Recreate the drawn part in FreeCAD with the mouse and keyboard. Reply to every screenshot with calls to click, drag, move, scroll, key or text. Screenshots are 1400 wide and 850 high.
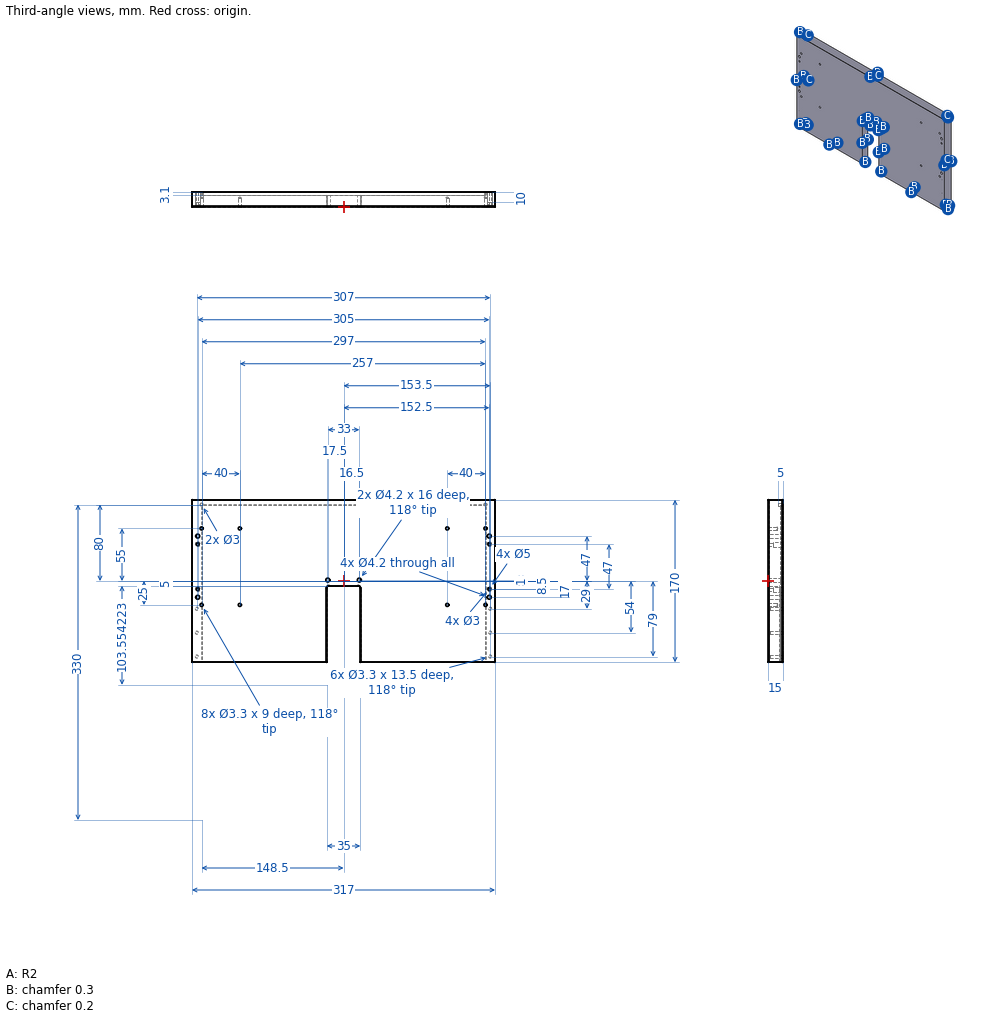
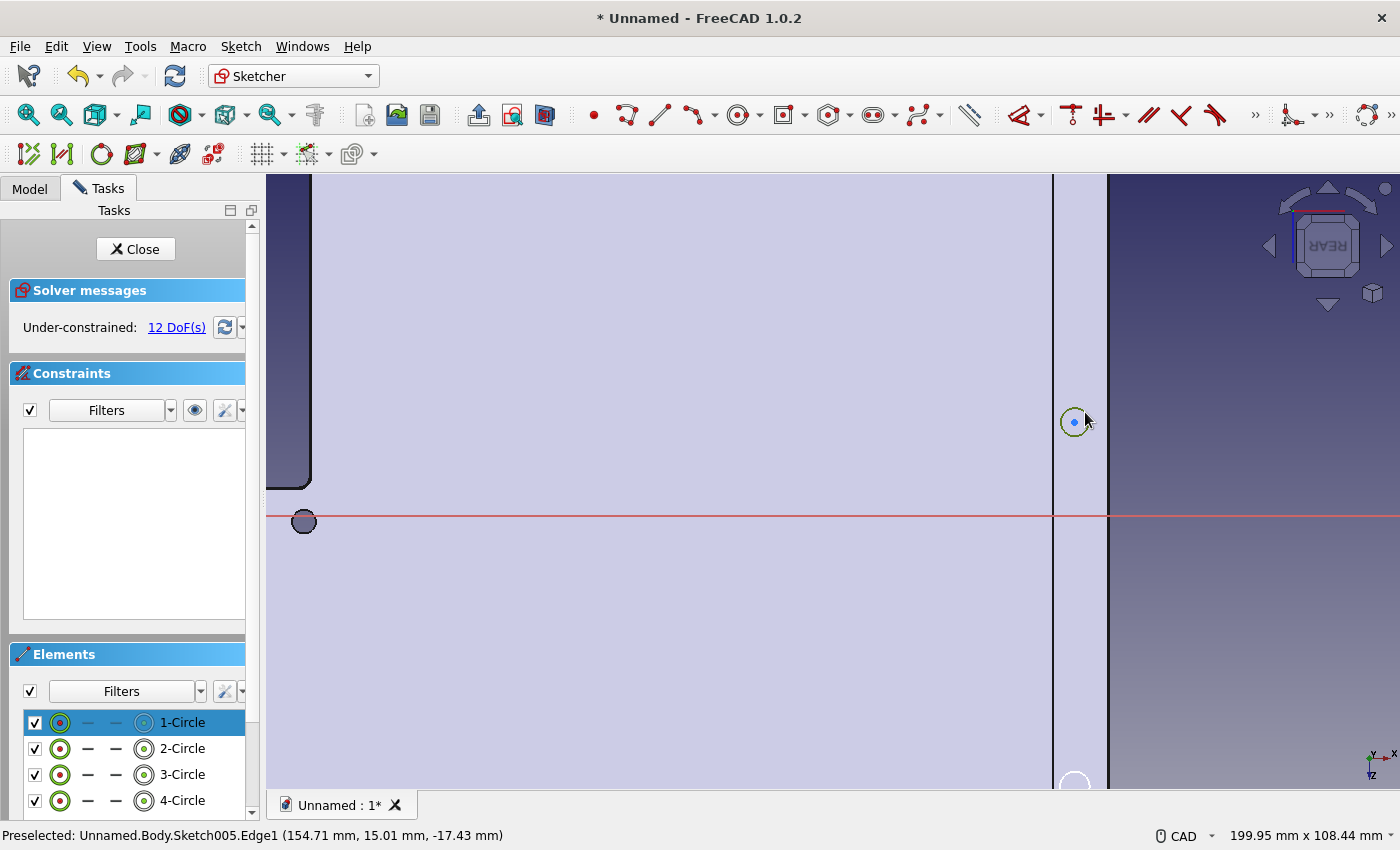
scroll(1087, 412, down, 5)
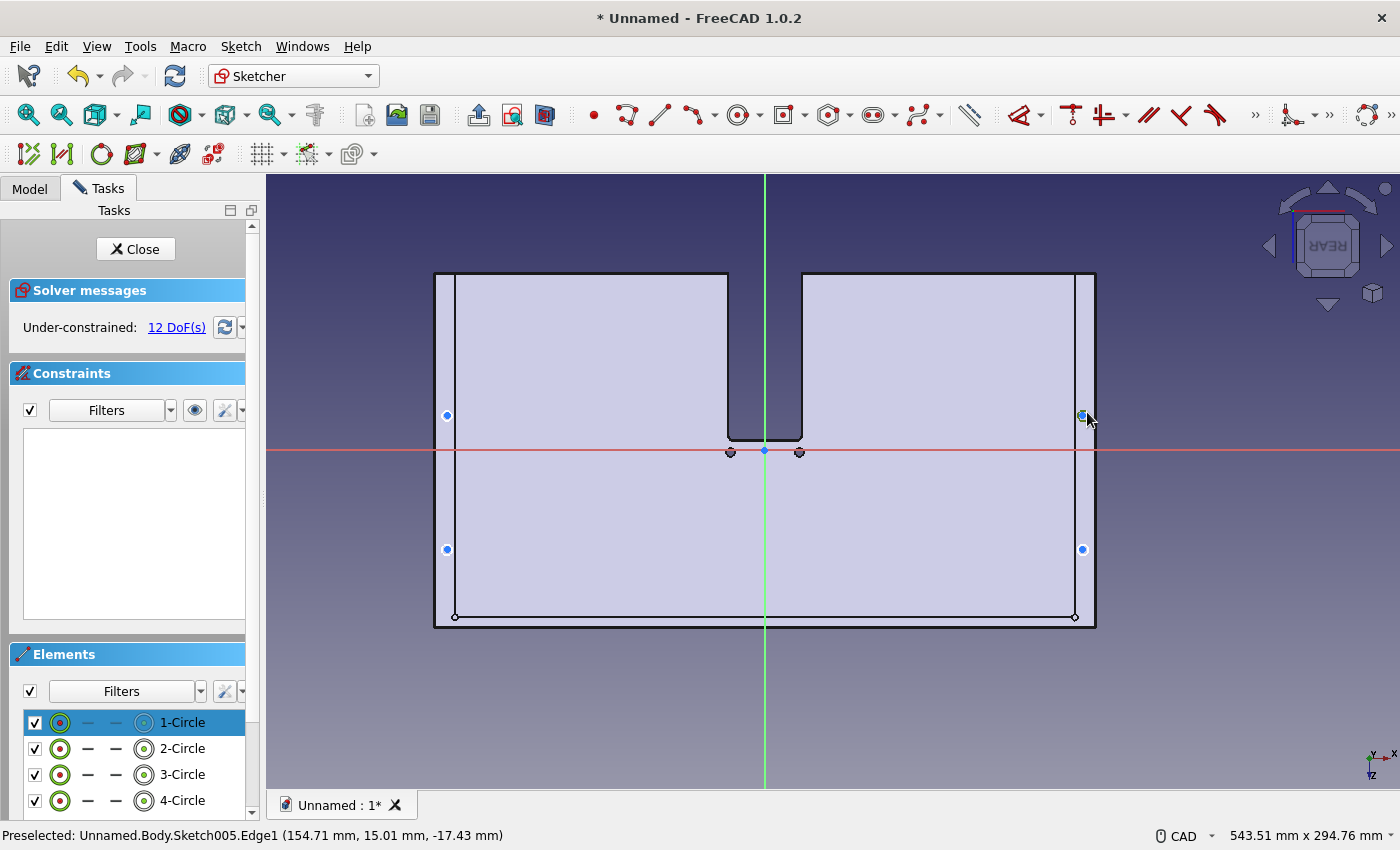
scroll(1087, 546, up, 5)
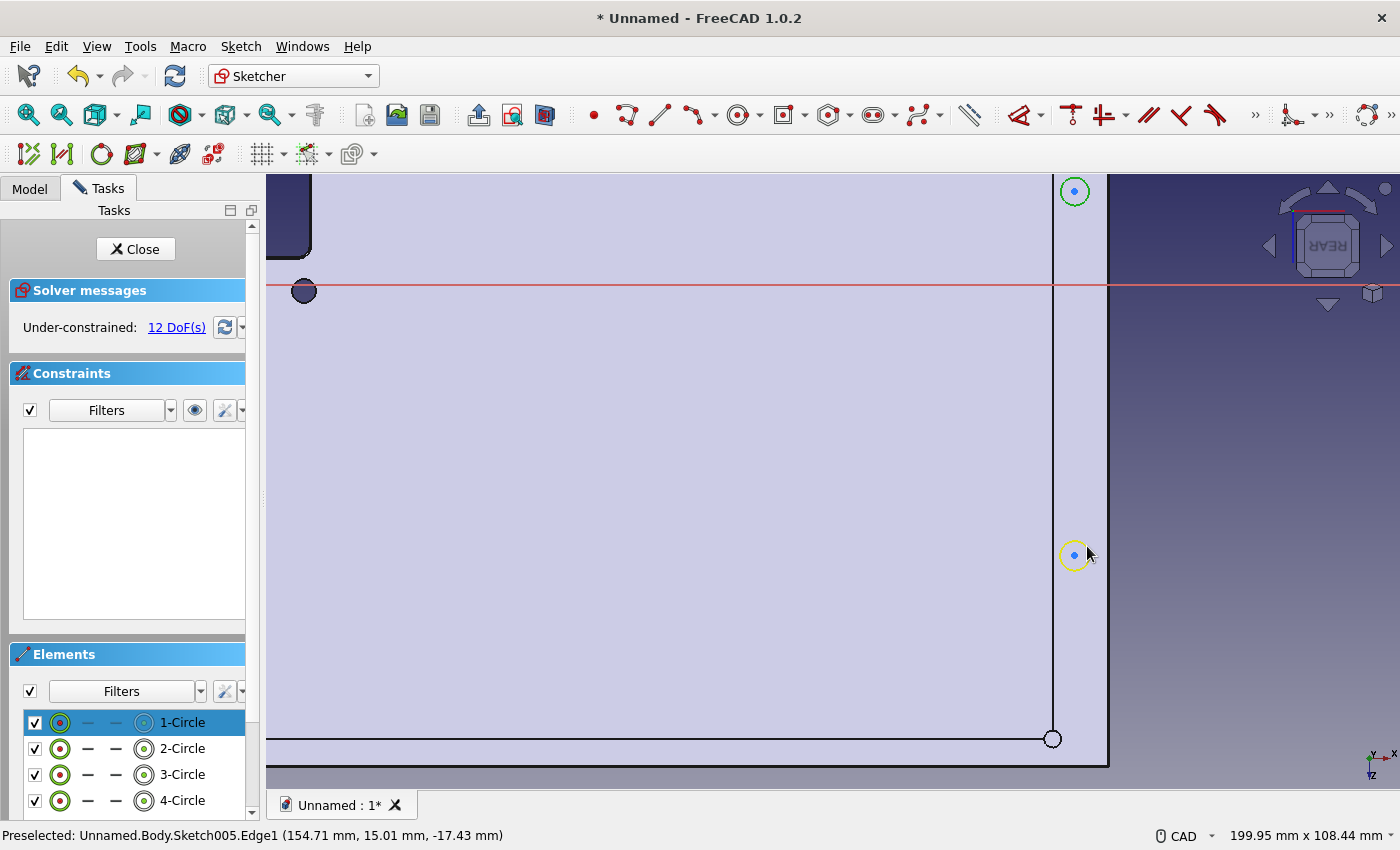
click(1085, 545)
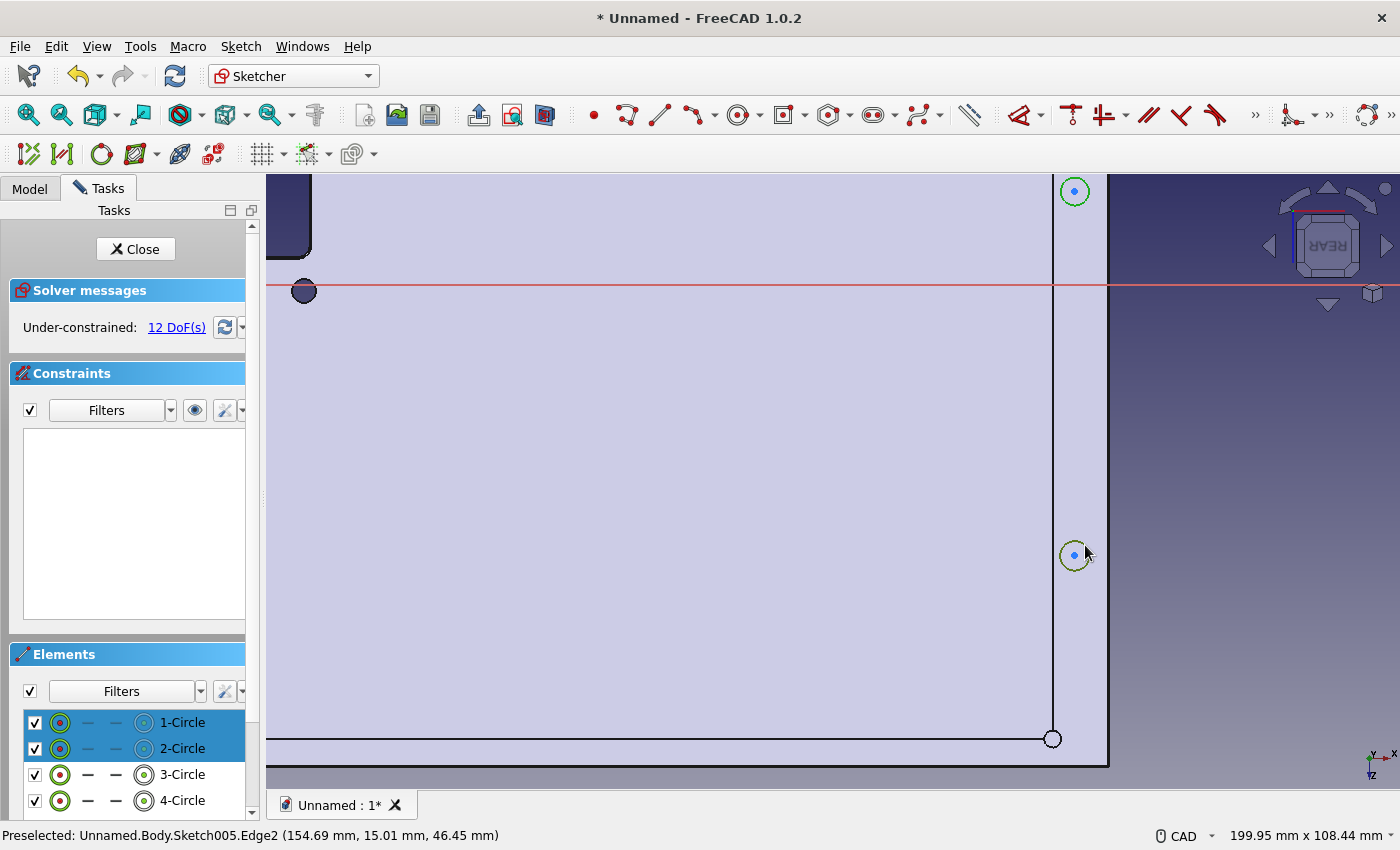
scroll(1087, 546, down, 5)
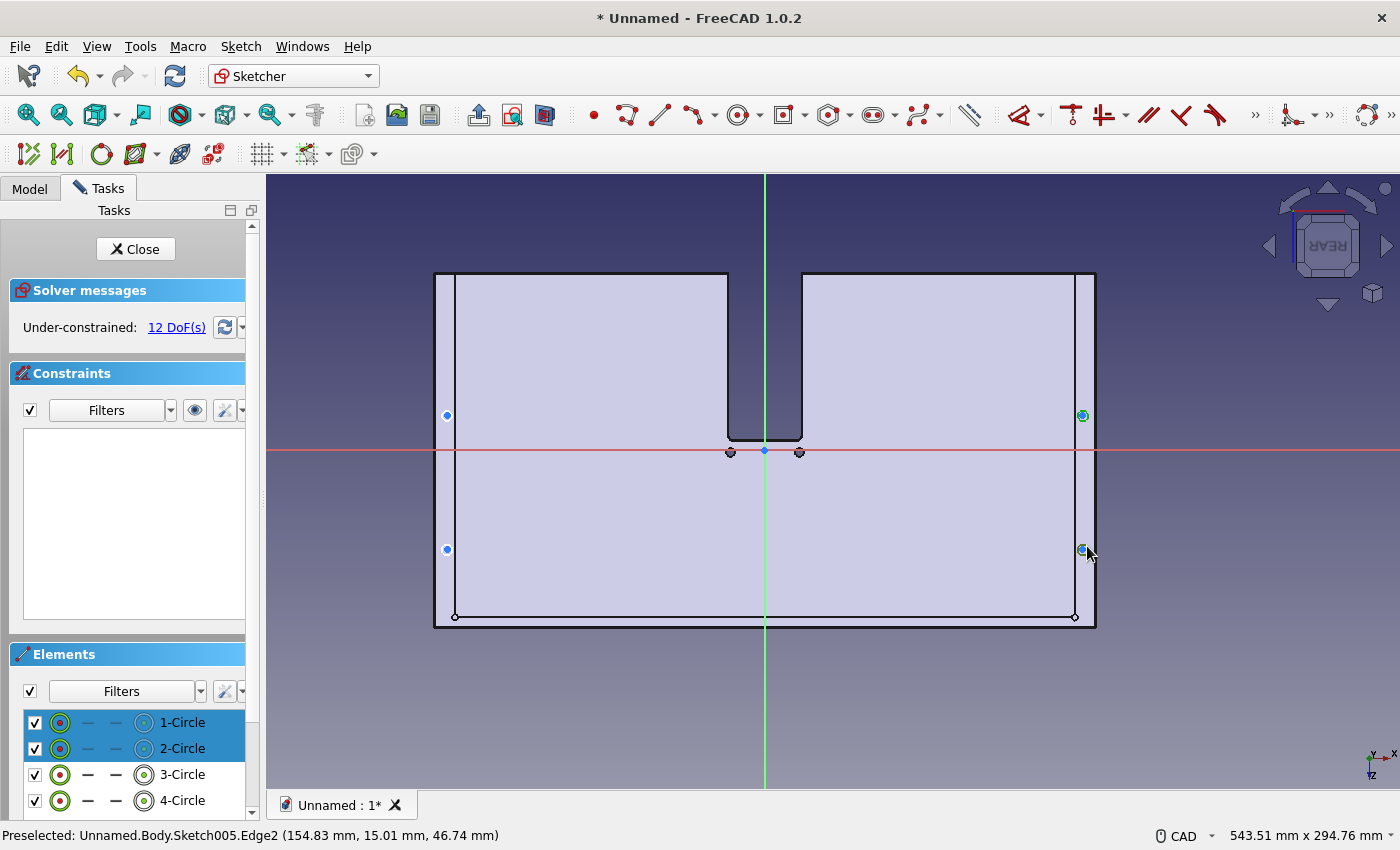
scroll(450, 413, up, 6)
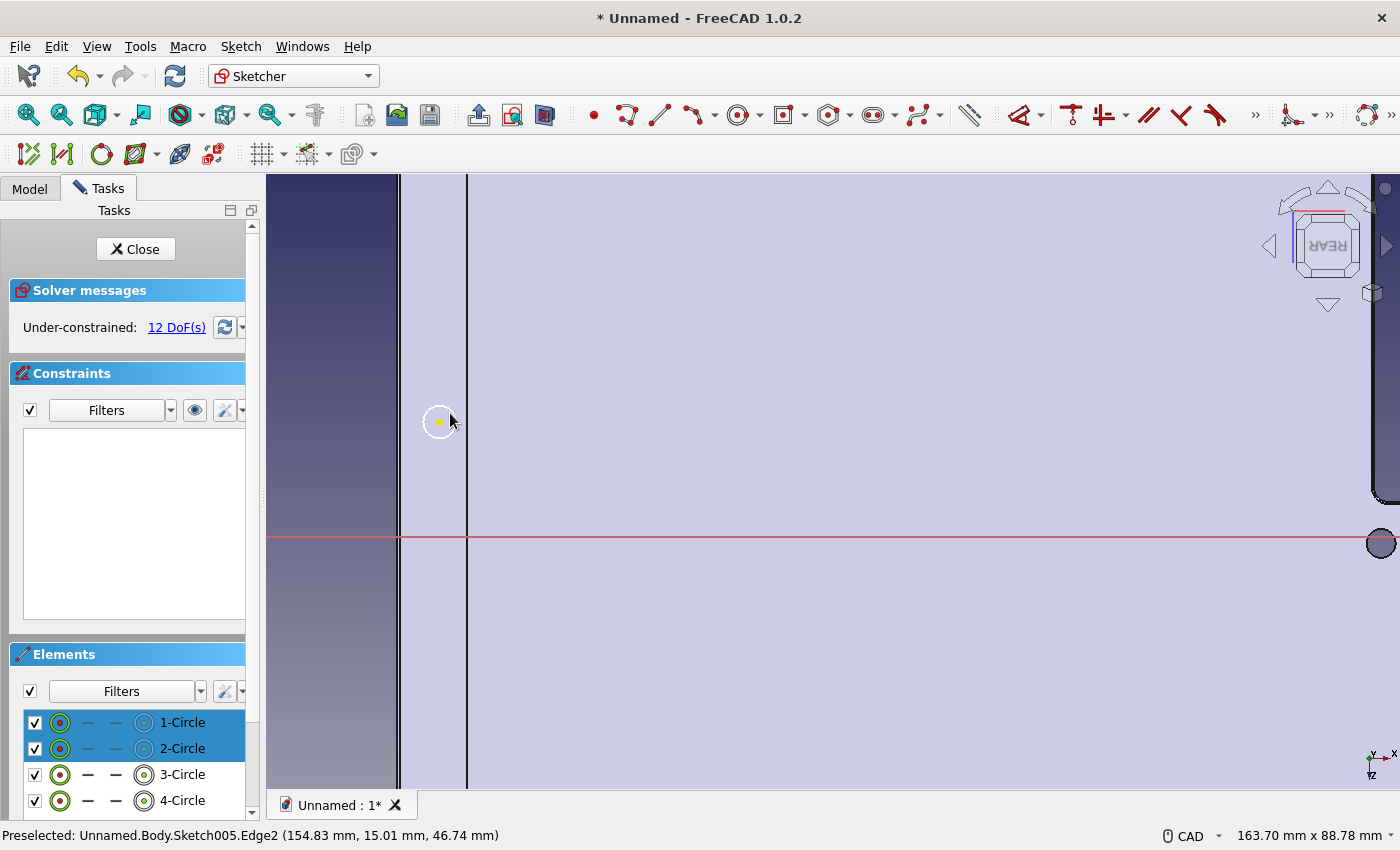
click(451, 411)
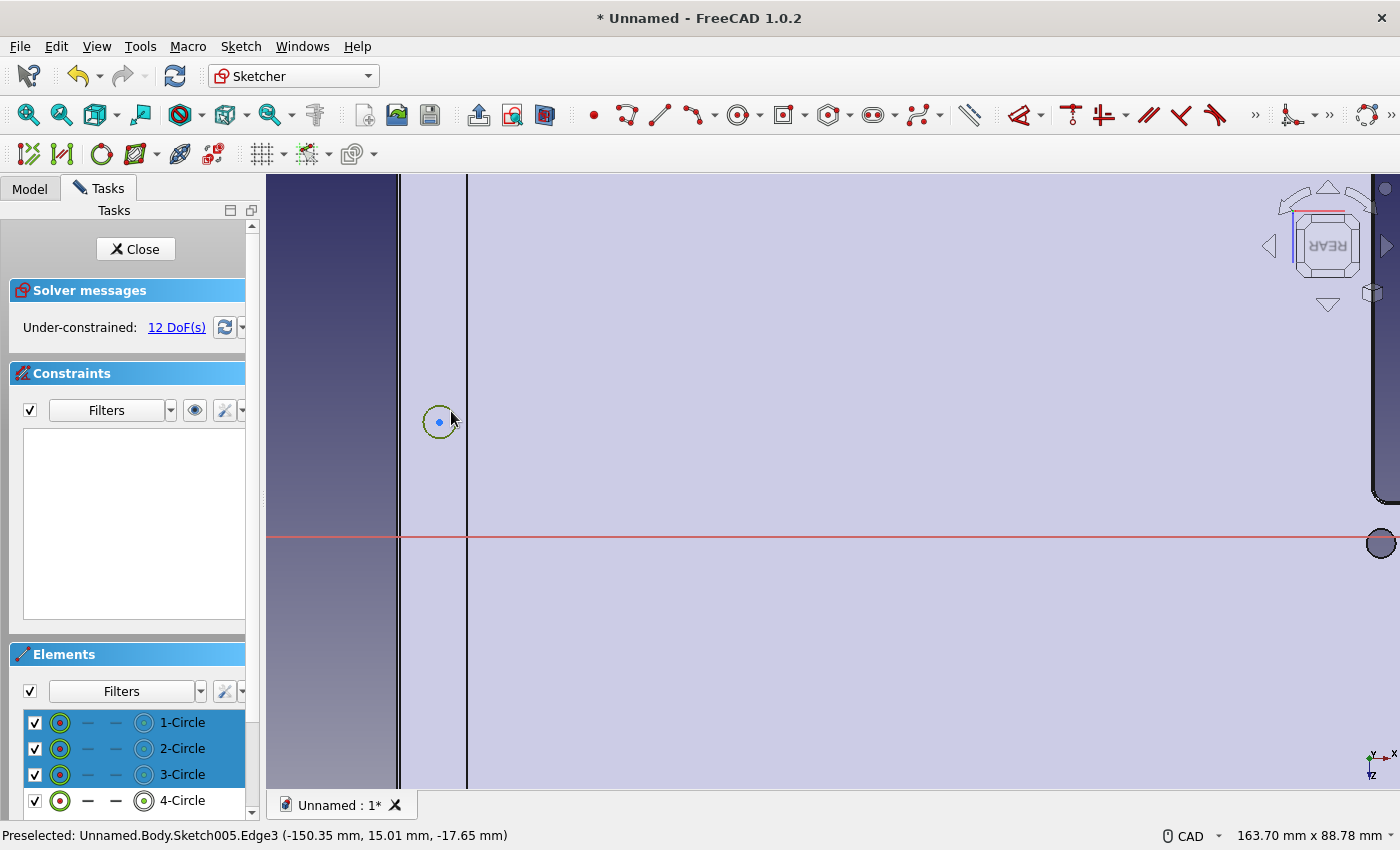
scroll(449, 413, down, 6)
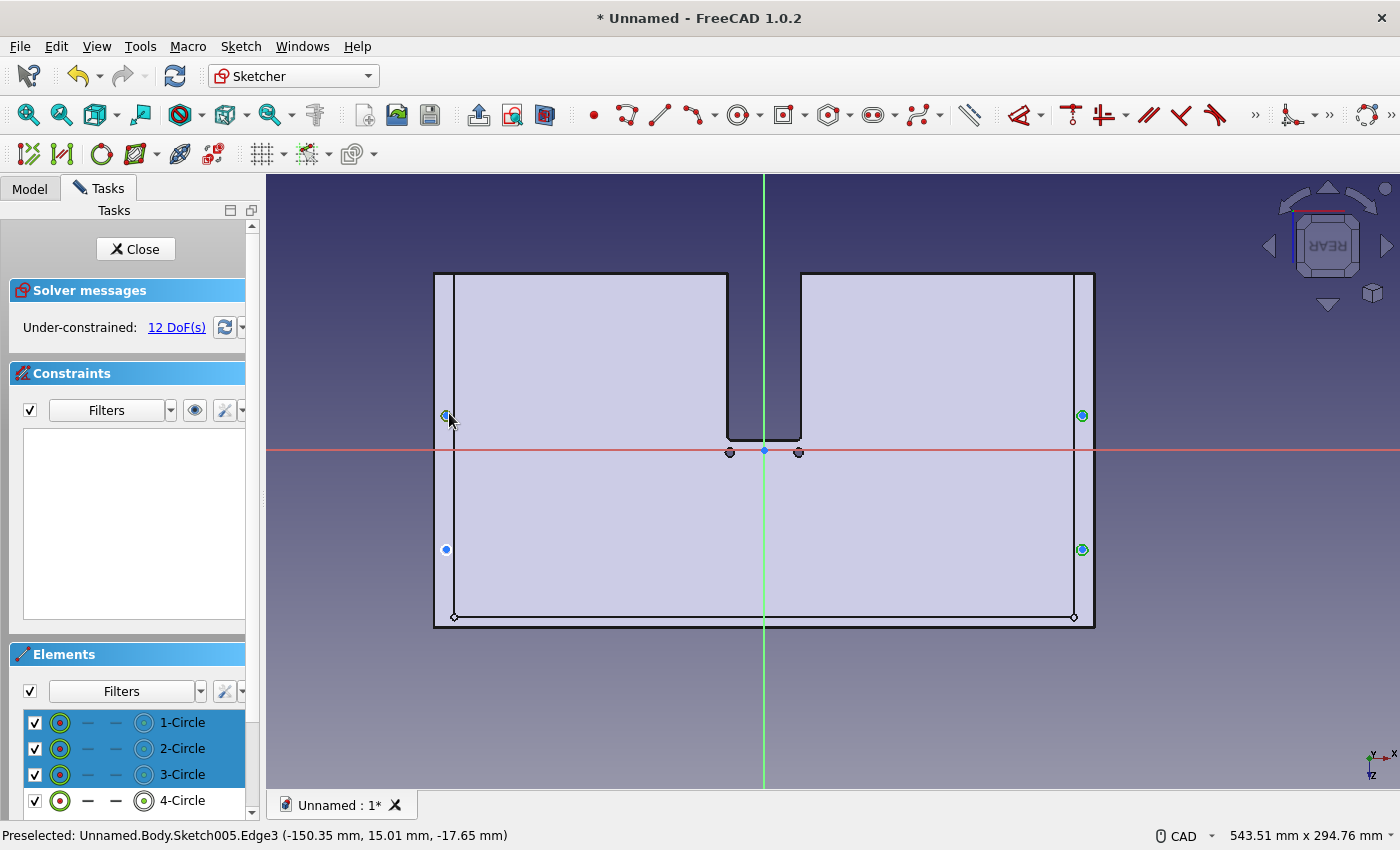
scroll(450, 546, up, 5)